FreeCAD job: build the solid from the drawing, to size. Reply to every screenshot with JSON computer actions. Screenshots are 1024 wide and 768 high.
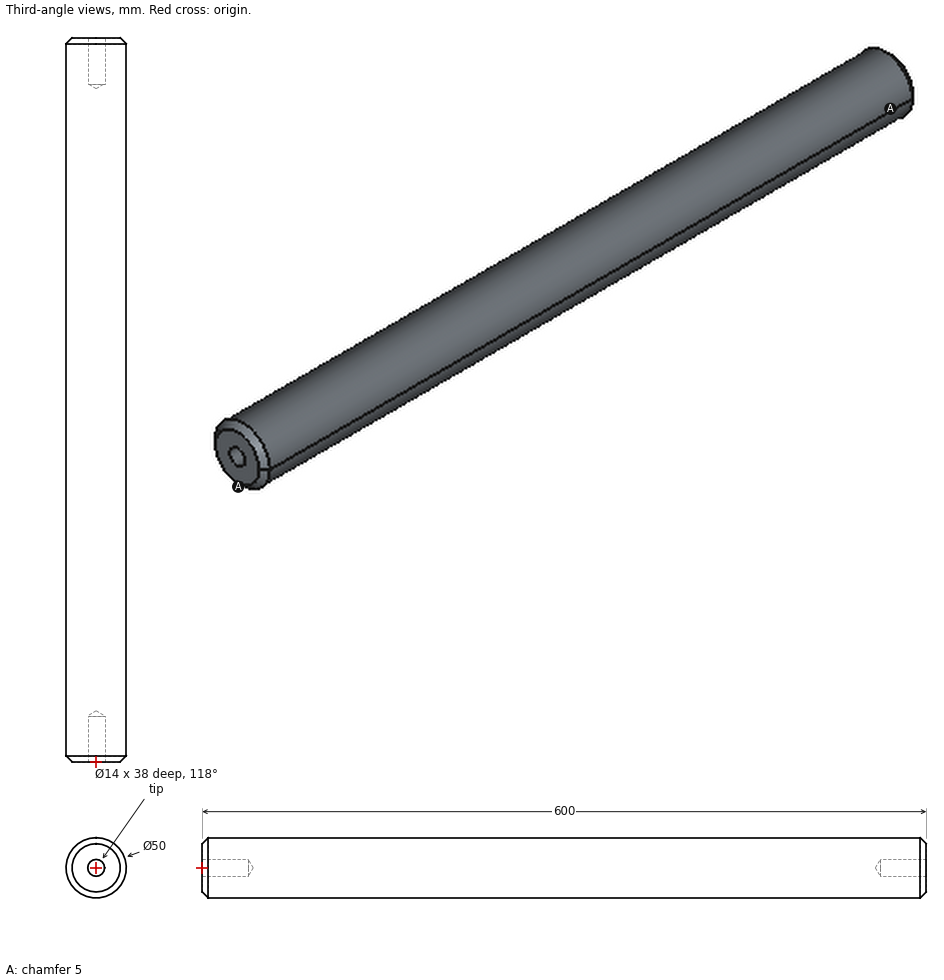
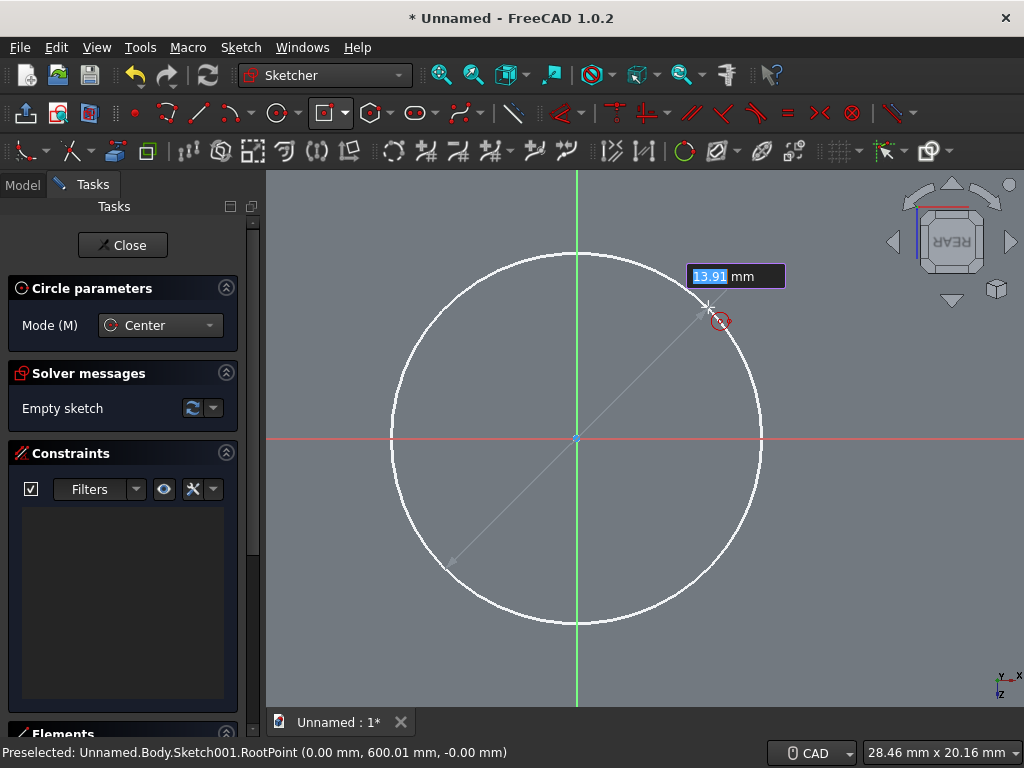
{"action": "type", "text": "14"}
{"action": "key", "text": "Return"}
{"action": "key", "text": "Escape"}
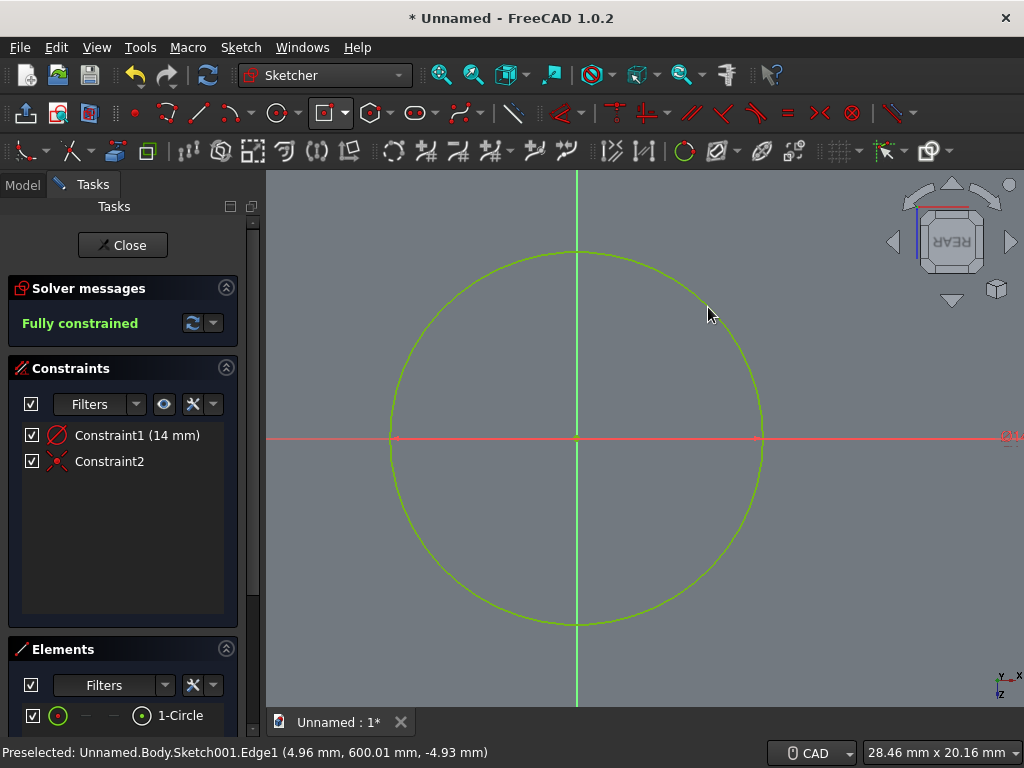
{"action": "left_click", "coordinate": [123, 245]}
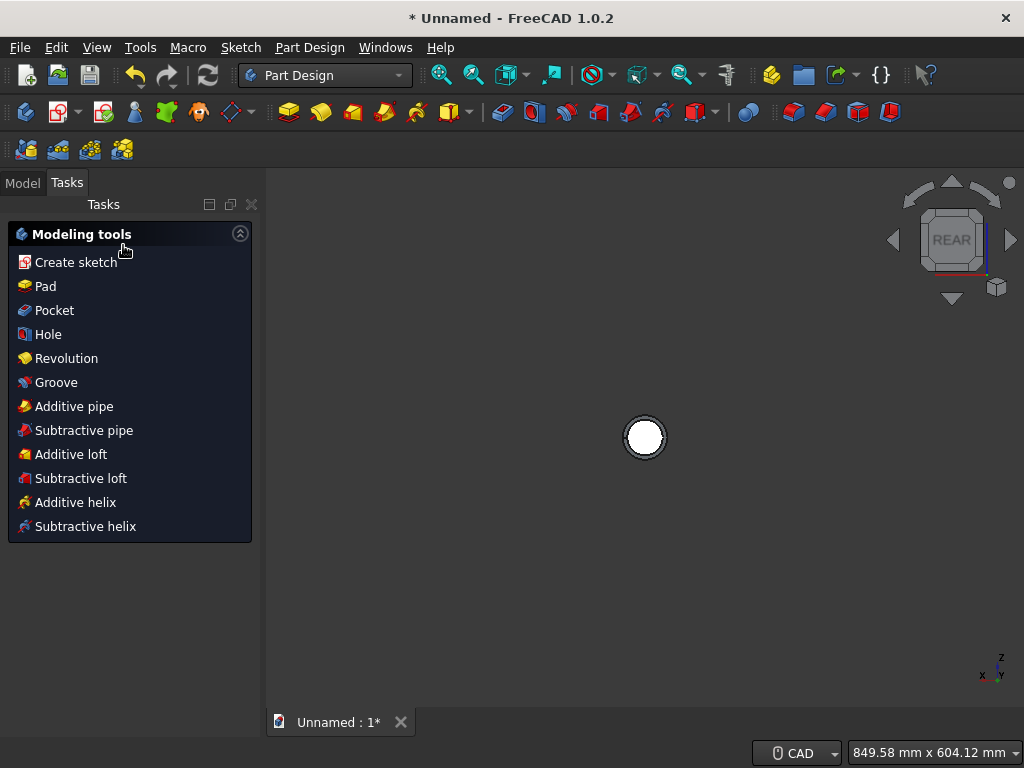
{"action": "left_click", "coordinate": [536, 112]}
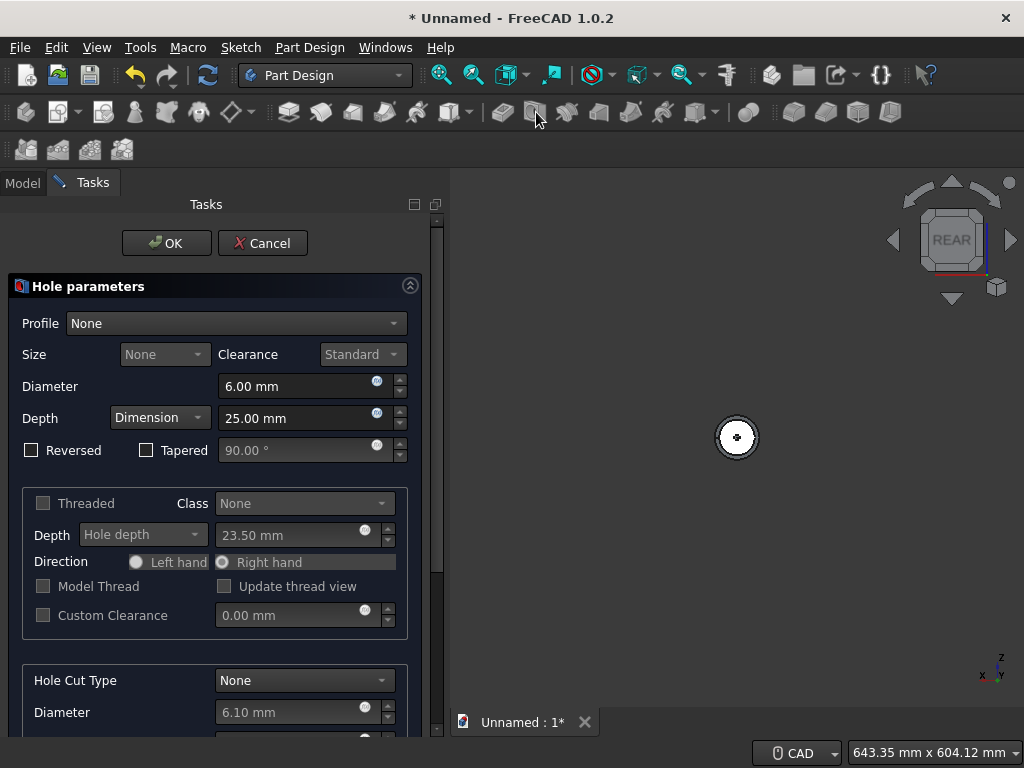
{"action": "triple_click", "coordinate": [305, 386]}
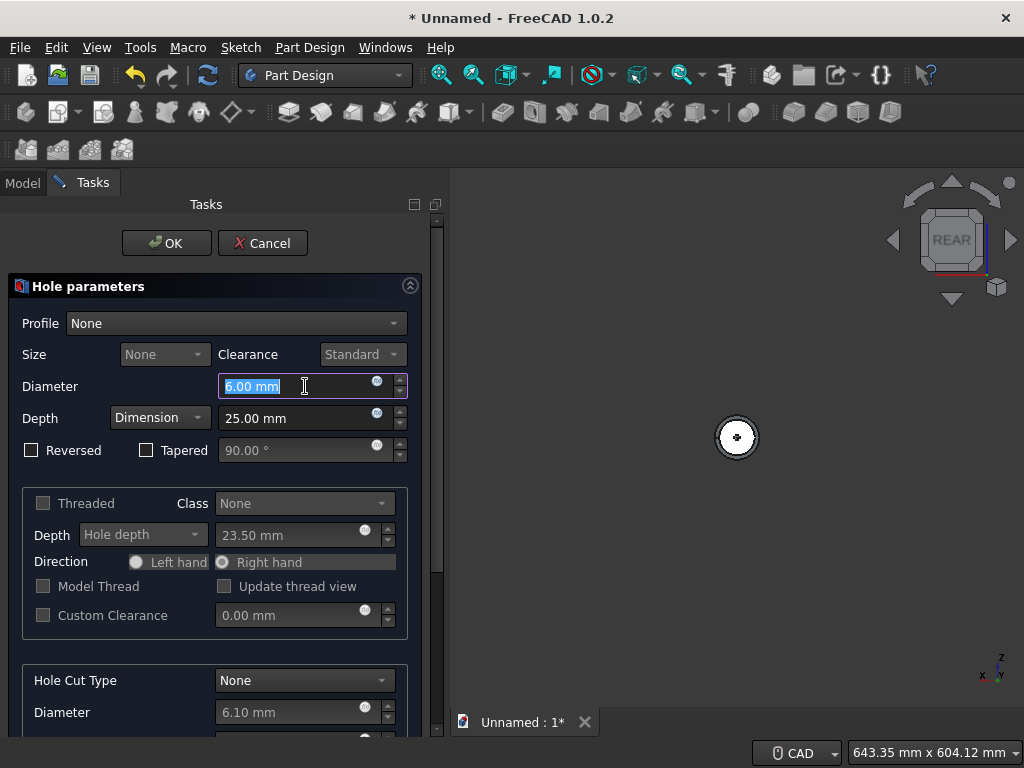
{"action": "type", "text": "14"}
{"action": "key", "text": "Tab"}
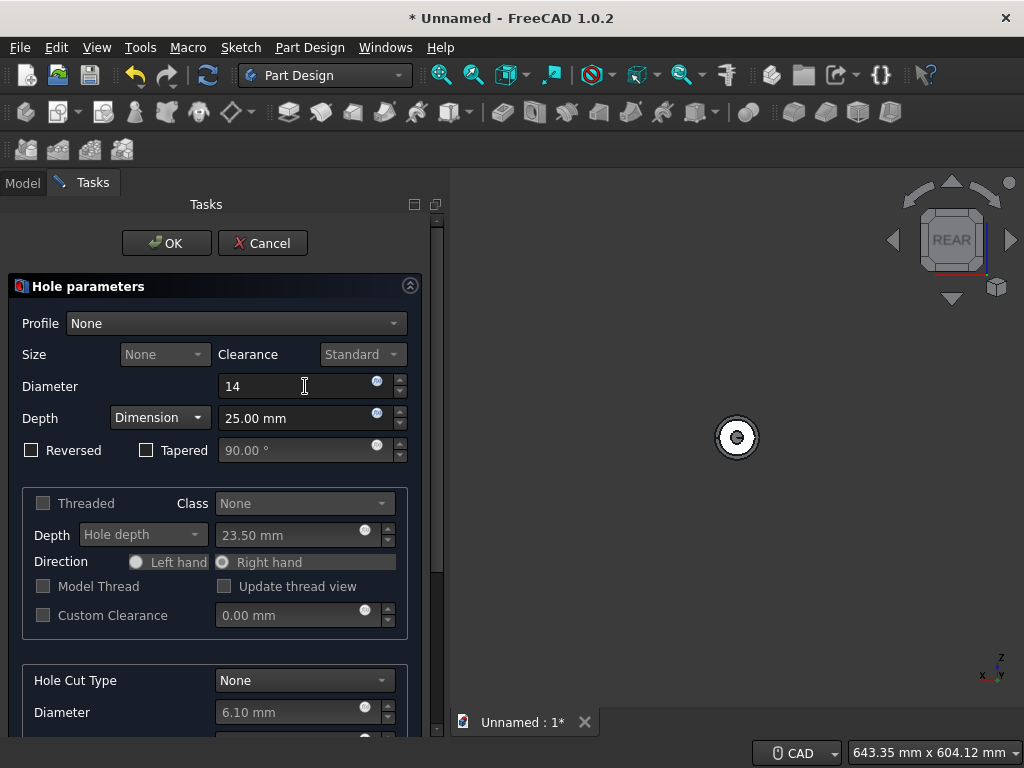
{"action": "triple_click", "coordinate": [305, 418]}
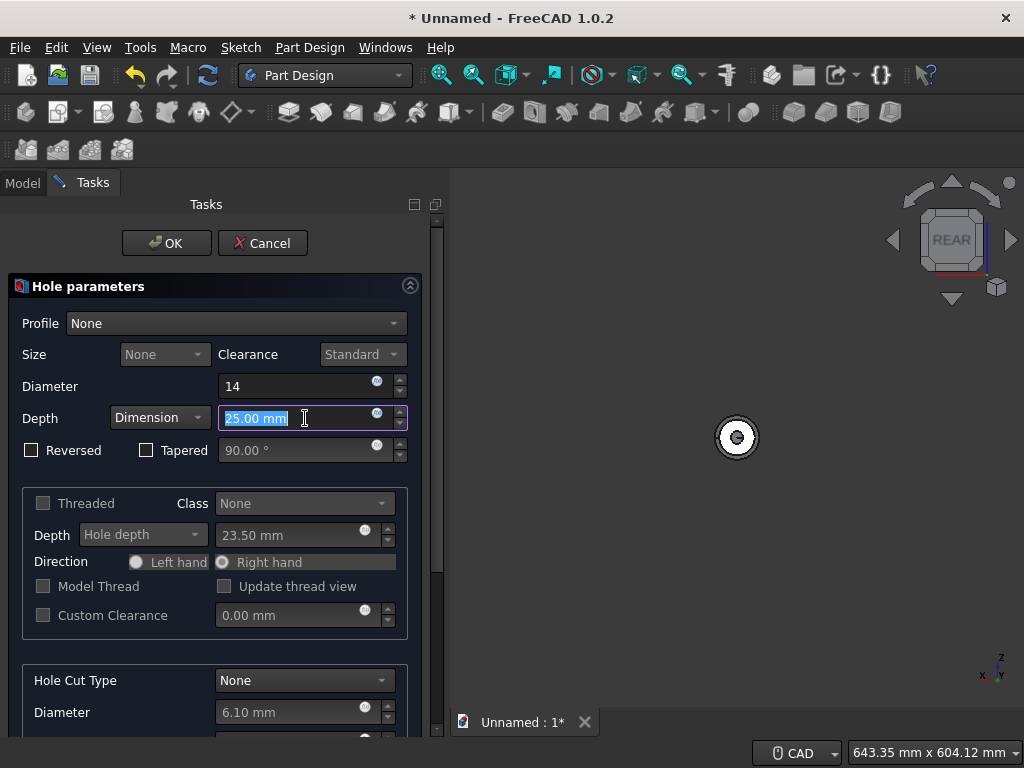
{"action": "type", "text": "38"}
{"action": "key", "text": "Tab"}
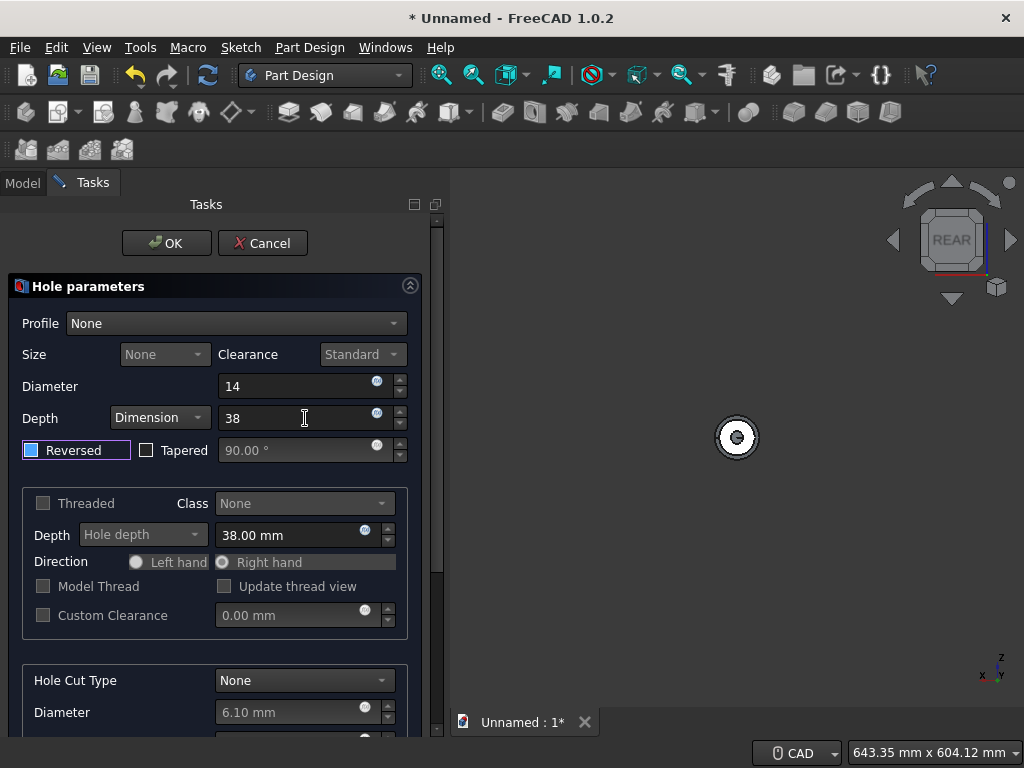
{"action": "left_click", "coordinate": [167, 243]}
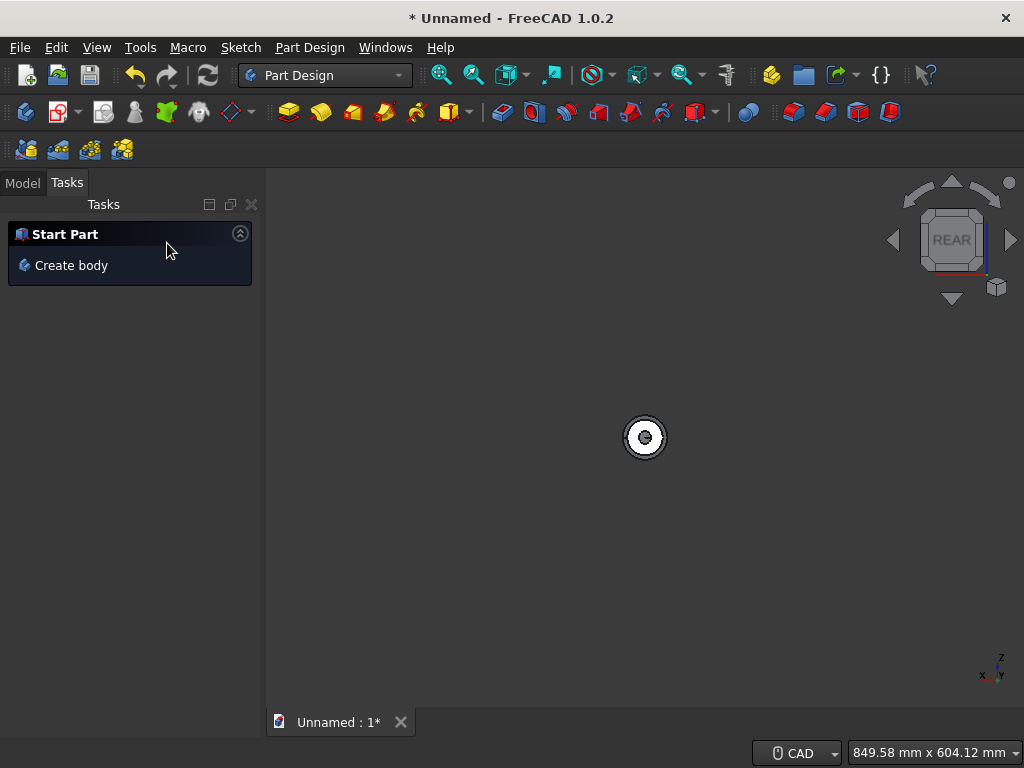
{"action": "left_click", "coordinate": [442, 76]}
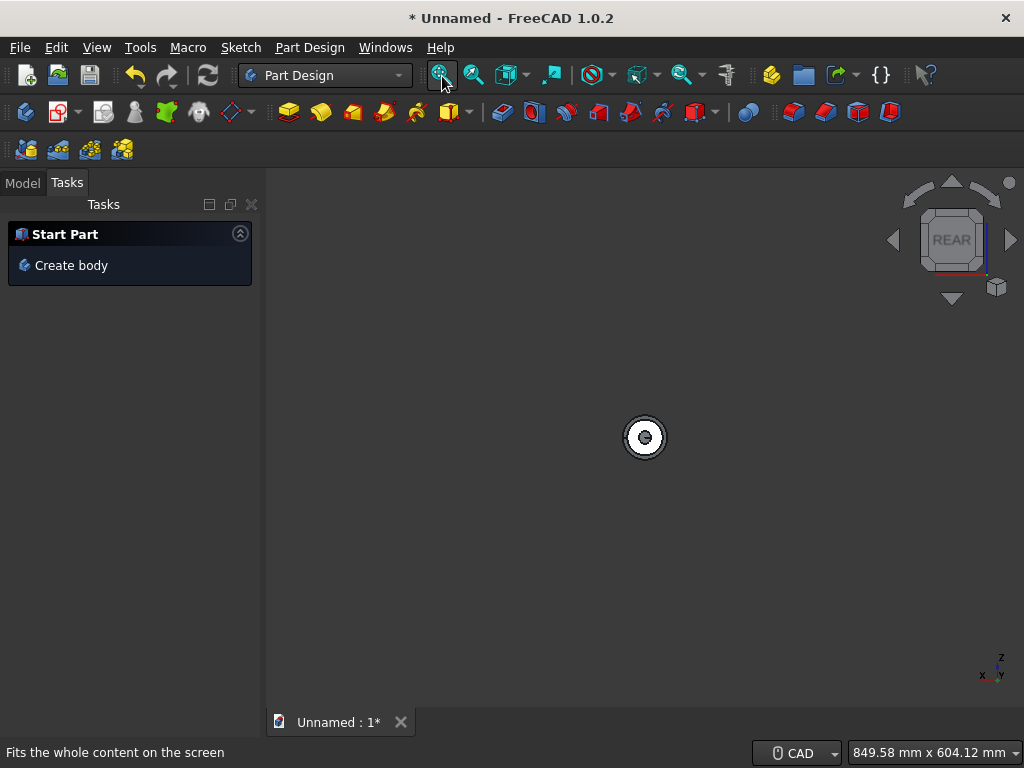
{"action": "left_click", "coordinate": [58, 112]}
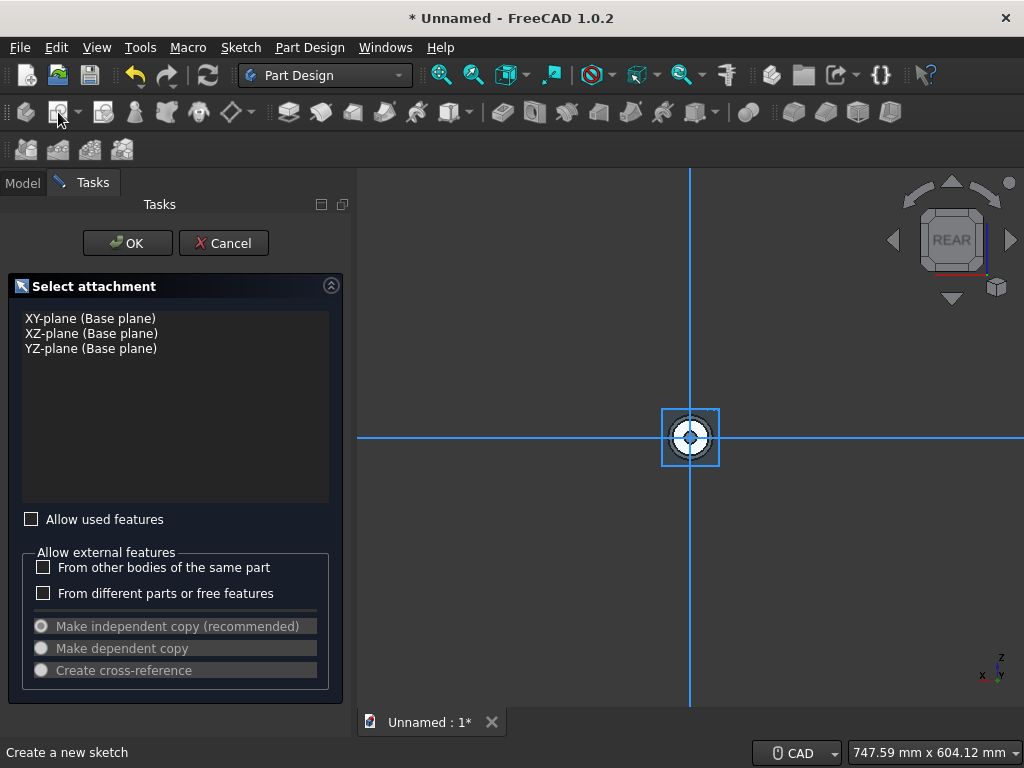
{"action": "left_click", "coordinate": [82, 334]}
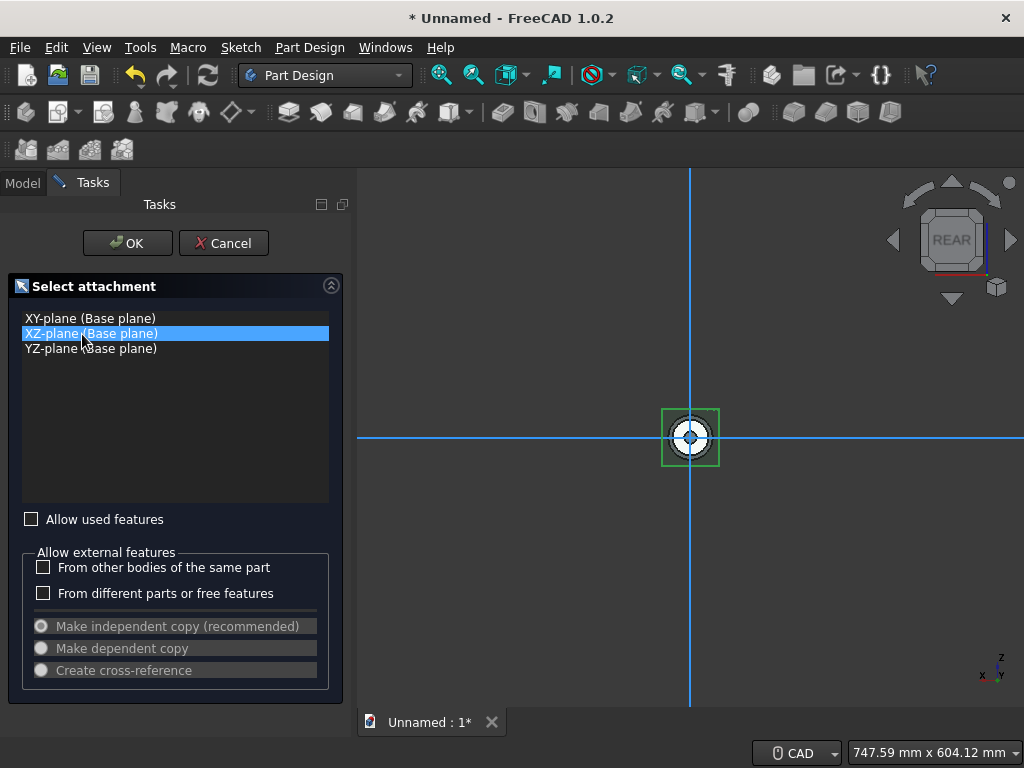
{"action": "left_click", "coordinate": [128, 243]}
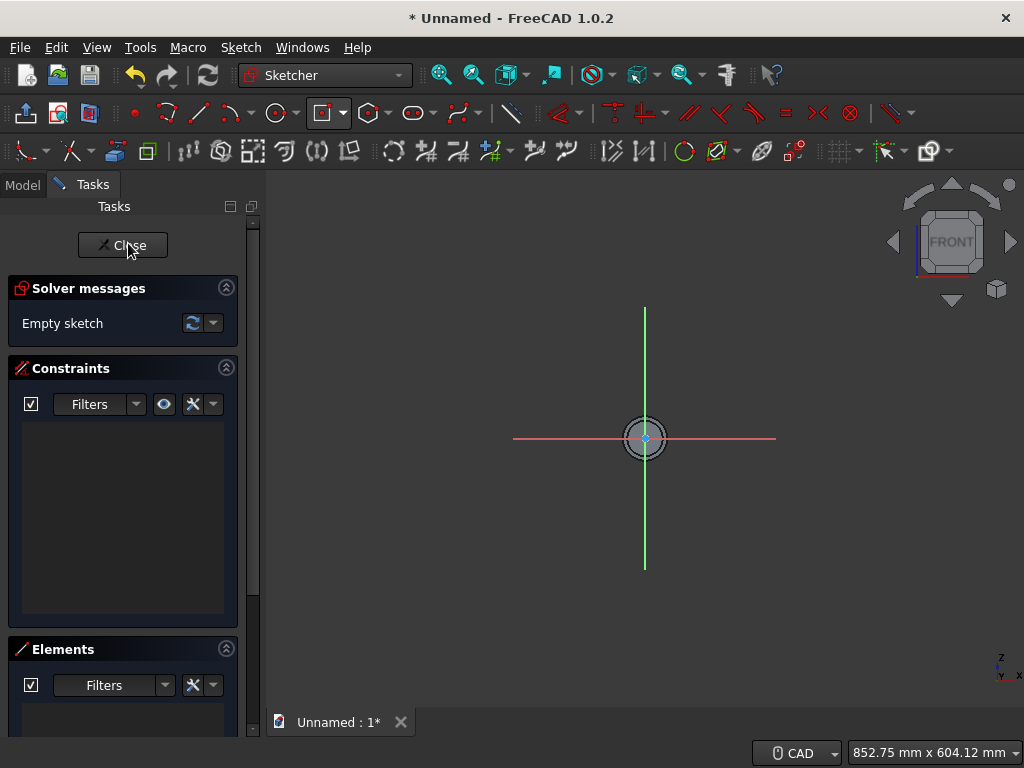
{"action": "scroll", "coordinate": [649, 439], "scroll_direction": "up", "scroll_amount": 15}